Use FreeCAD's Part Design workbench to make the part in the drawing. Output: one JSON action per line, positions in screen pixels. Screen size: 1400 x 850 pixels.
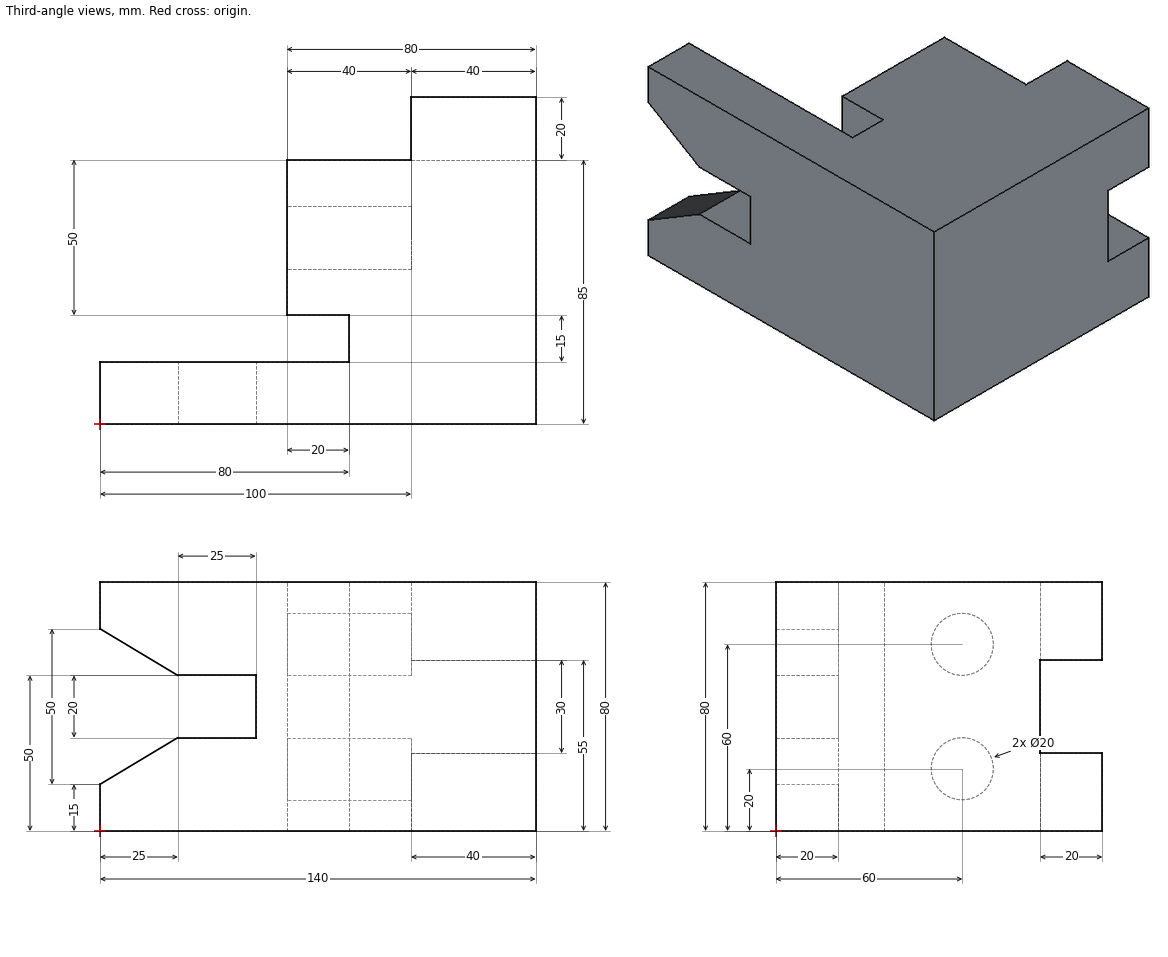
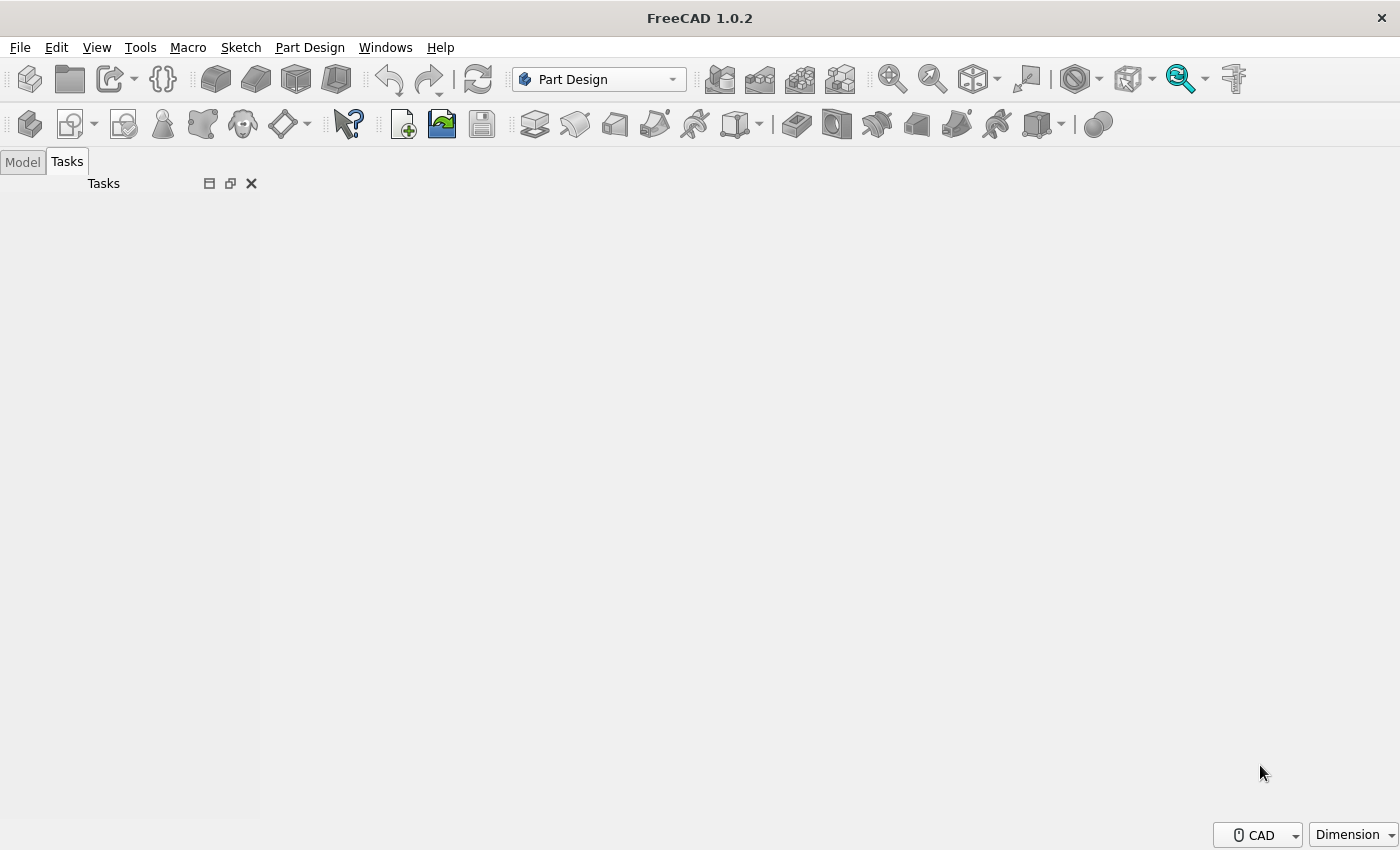
{"action": "key", "text": "ctrl+n"}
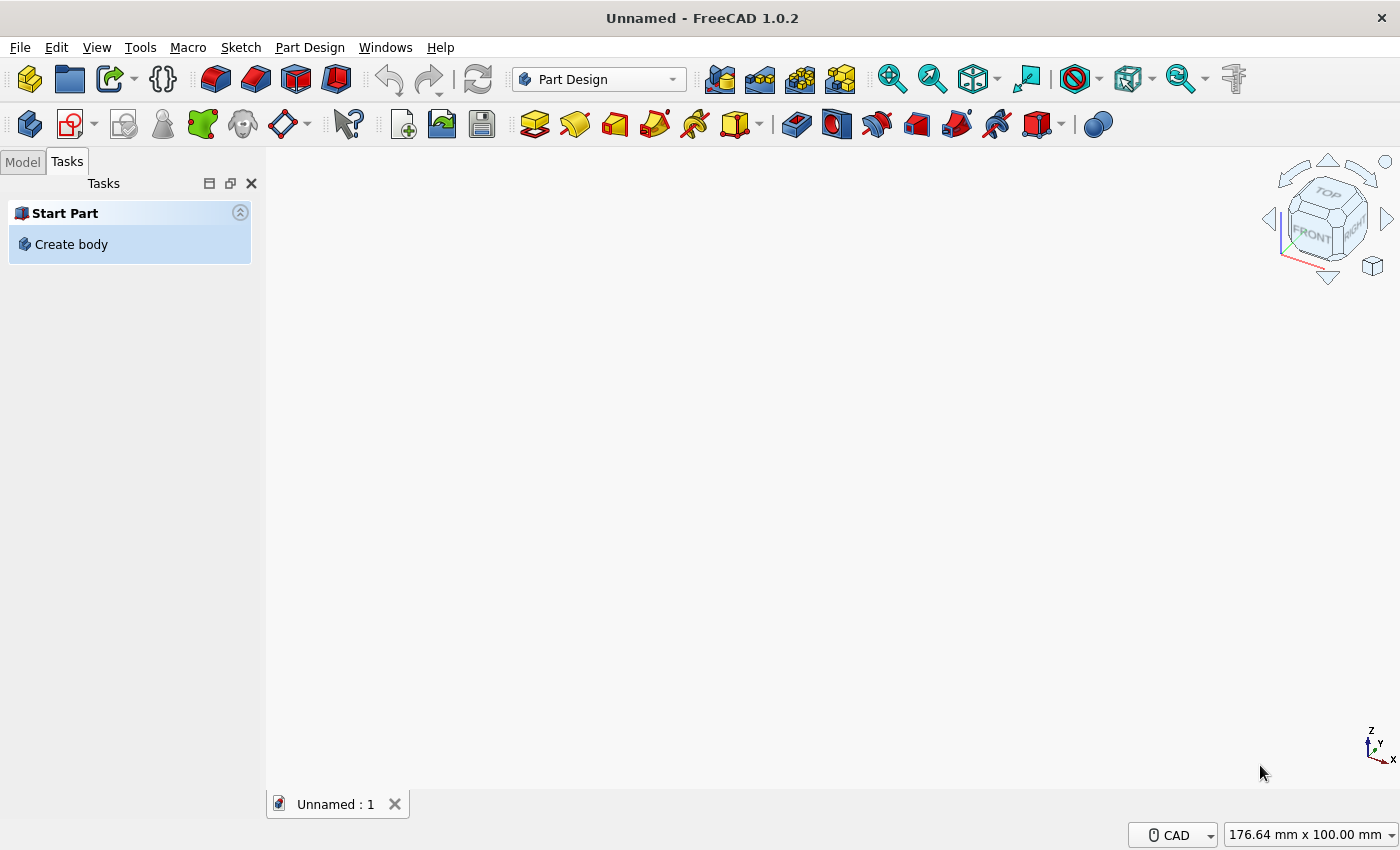
{"action": "left_click", "coordinate": [70, 124]}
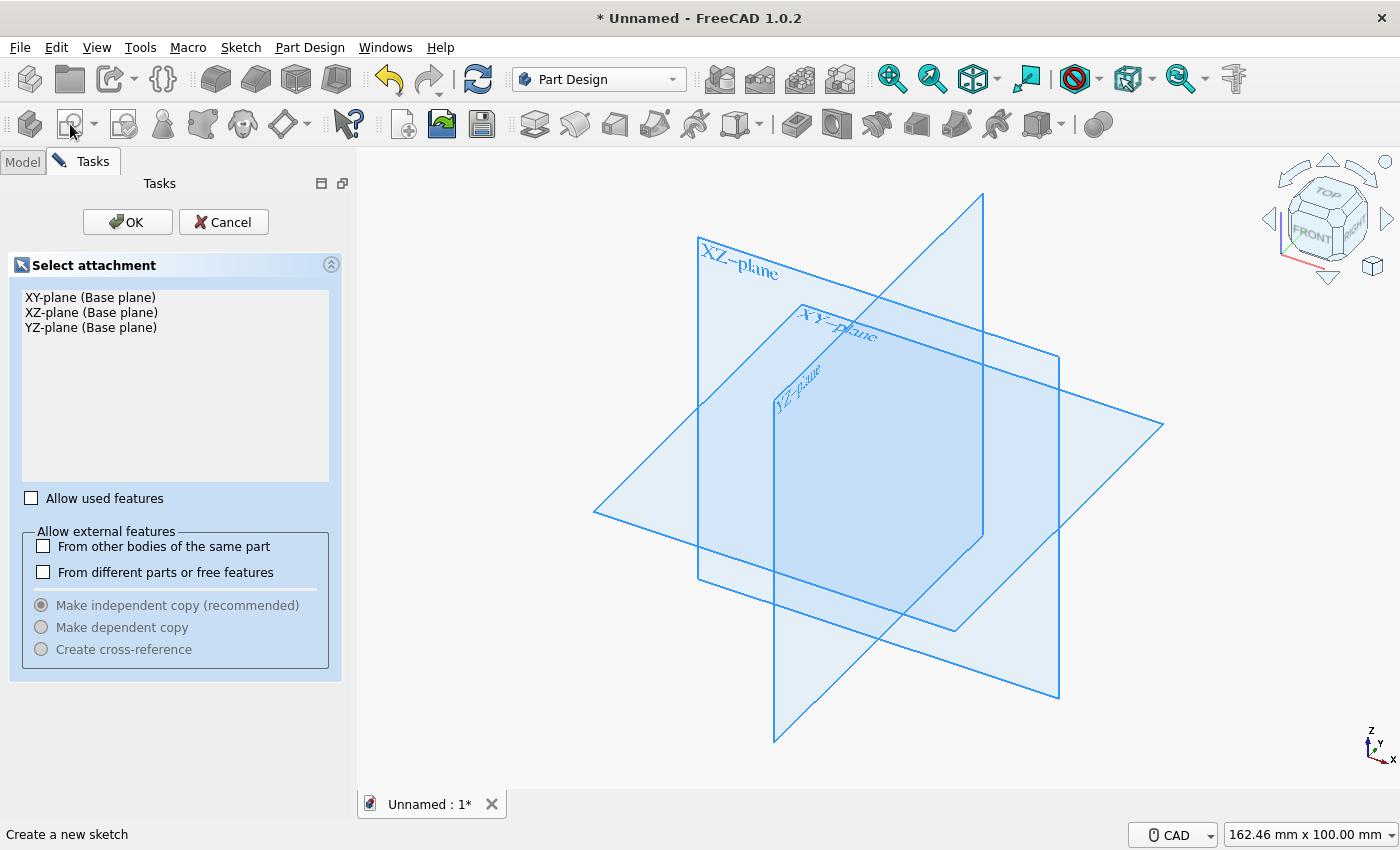
{"action": "left_click", "coordinate": [82, 298]}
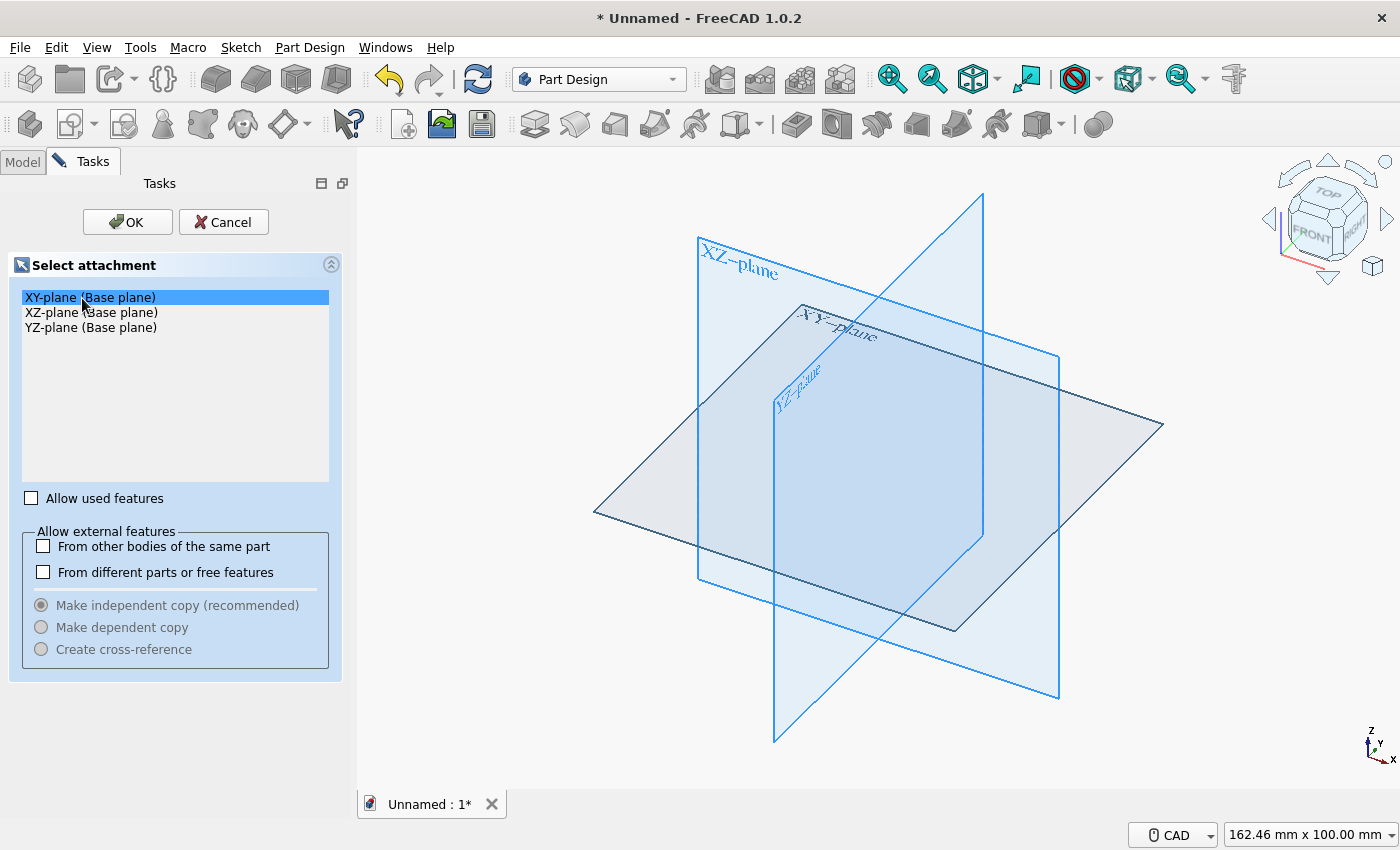
{"action": "left_click", "coordinate": [128, 222]}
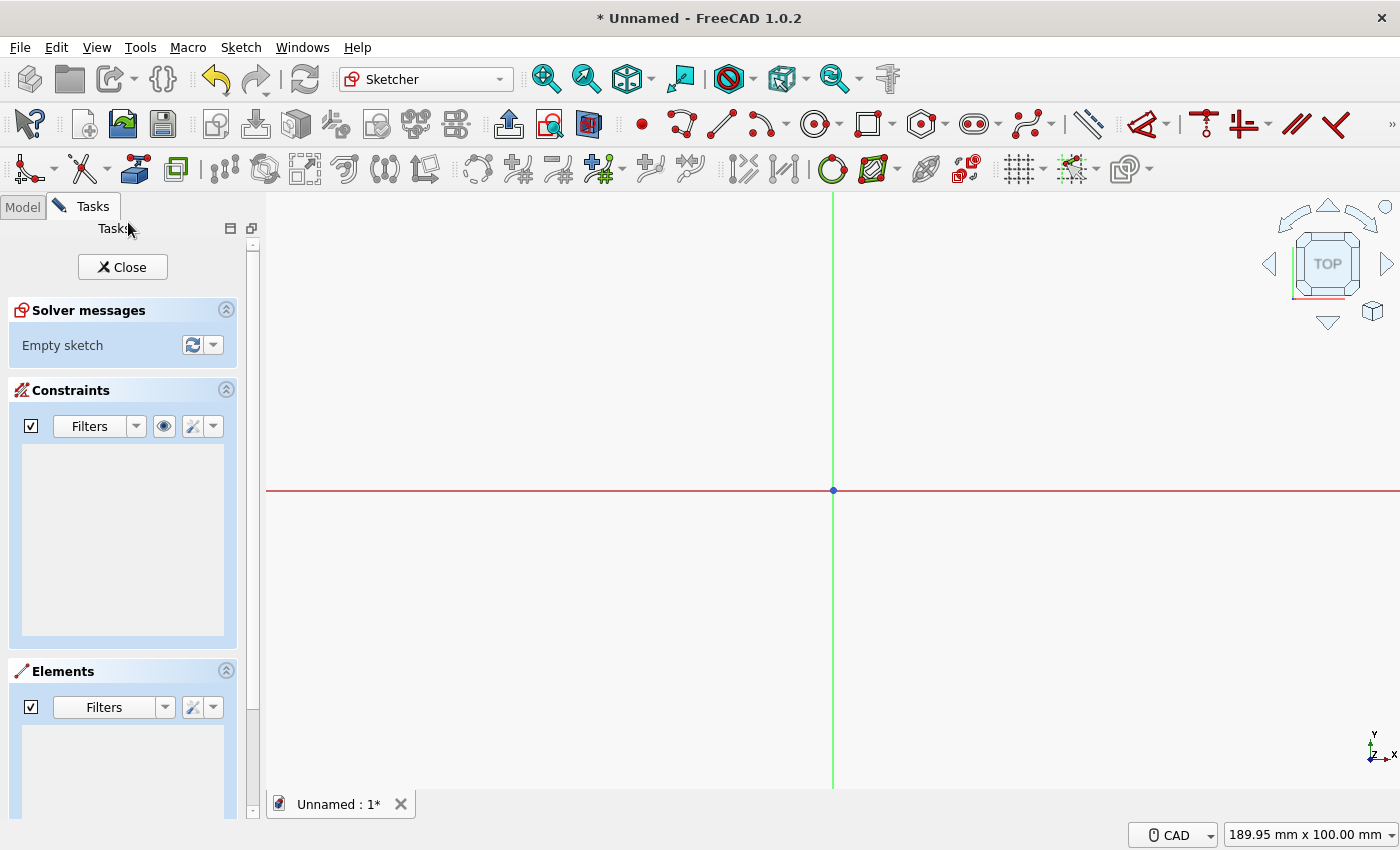
{"action": "scroll", "coordinate": [294, 761], "scroll_direction": "down", "scroll_amount": 3}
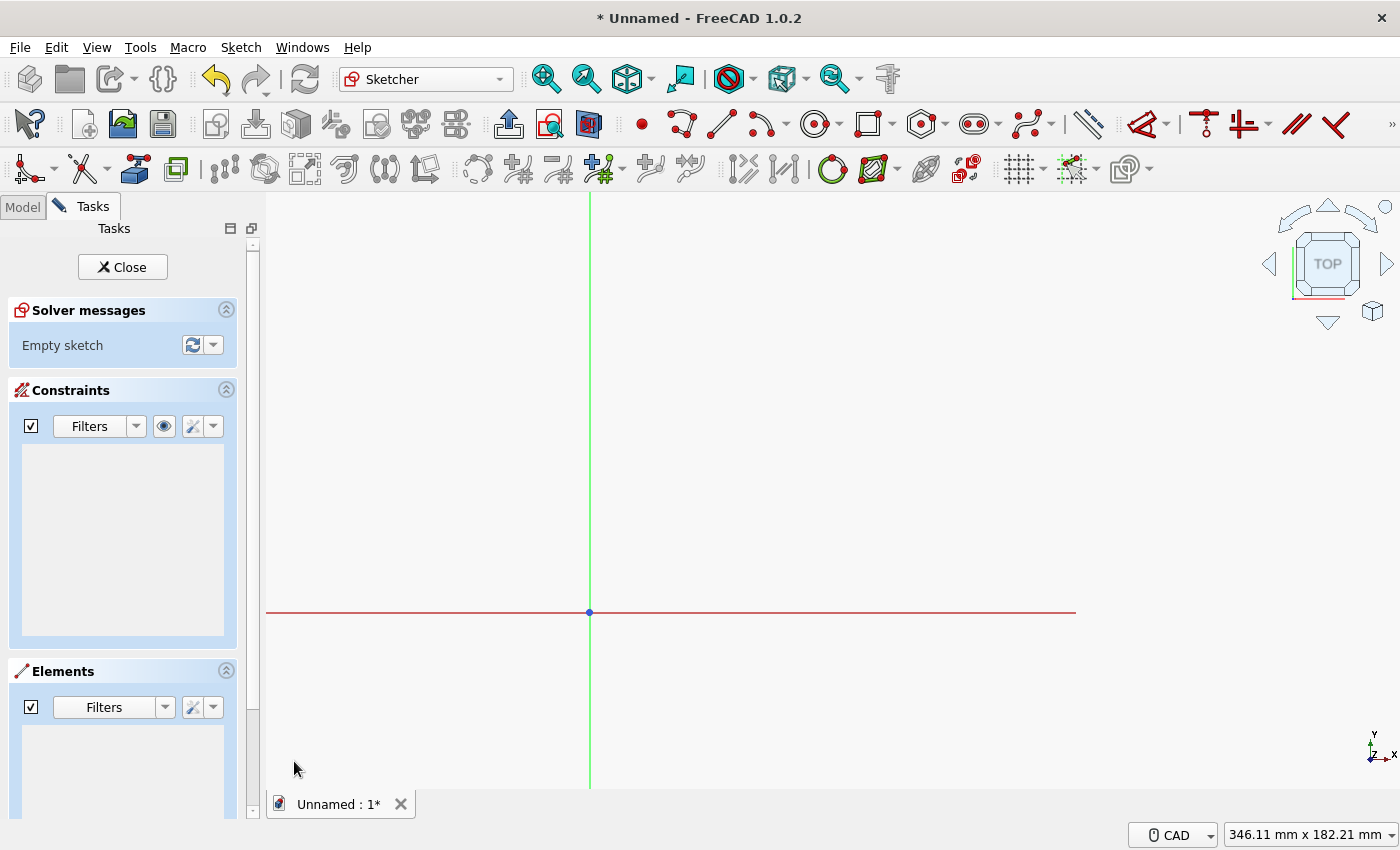
{"action": "scroll", "coordinate": [930, 440], "scroll_direction": "up", "scroll_amount": 2}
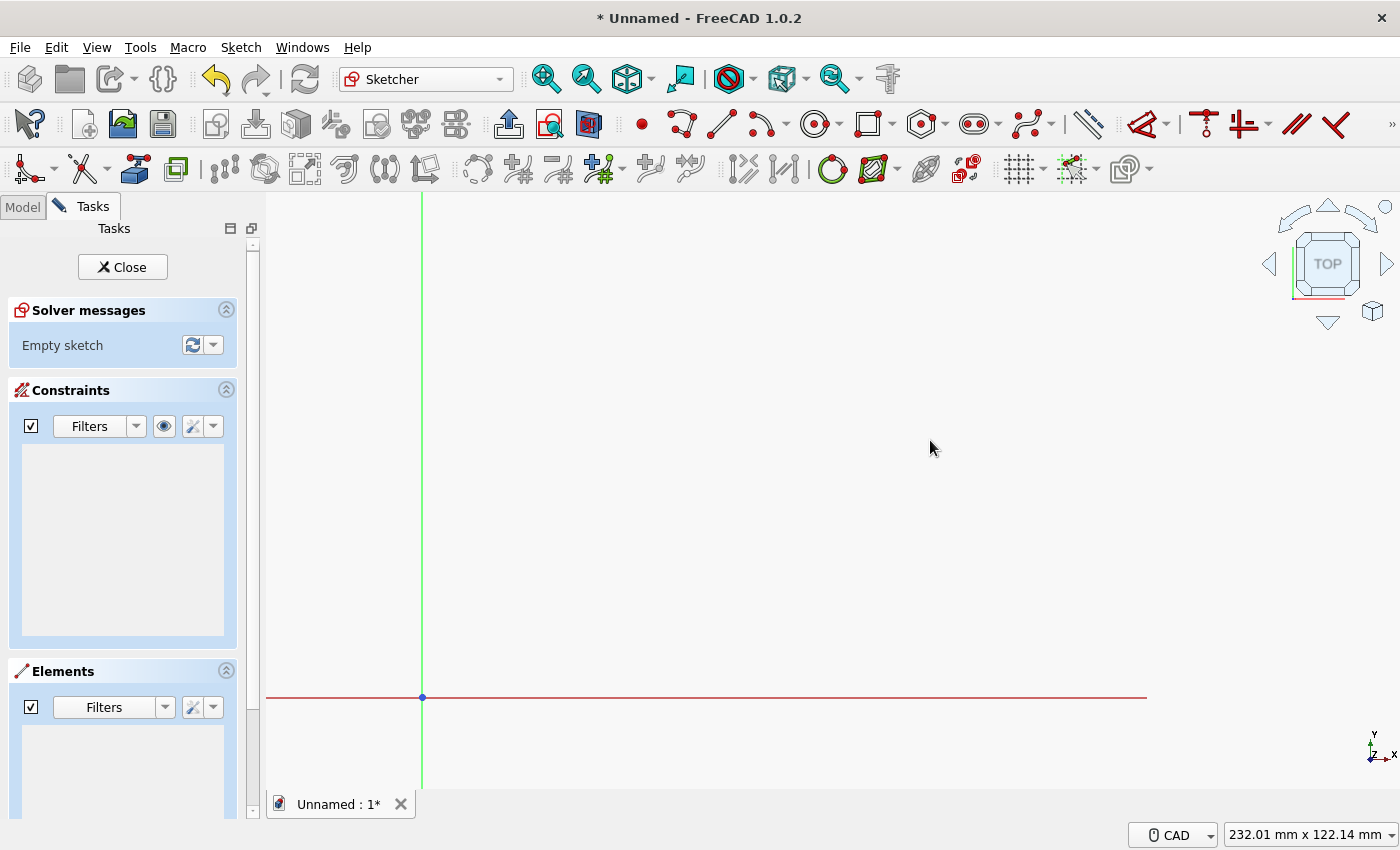
{"action": "left_click", "coordinate": [682, 124]}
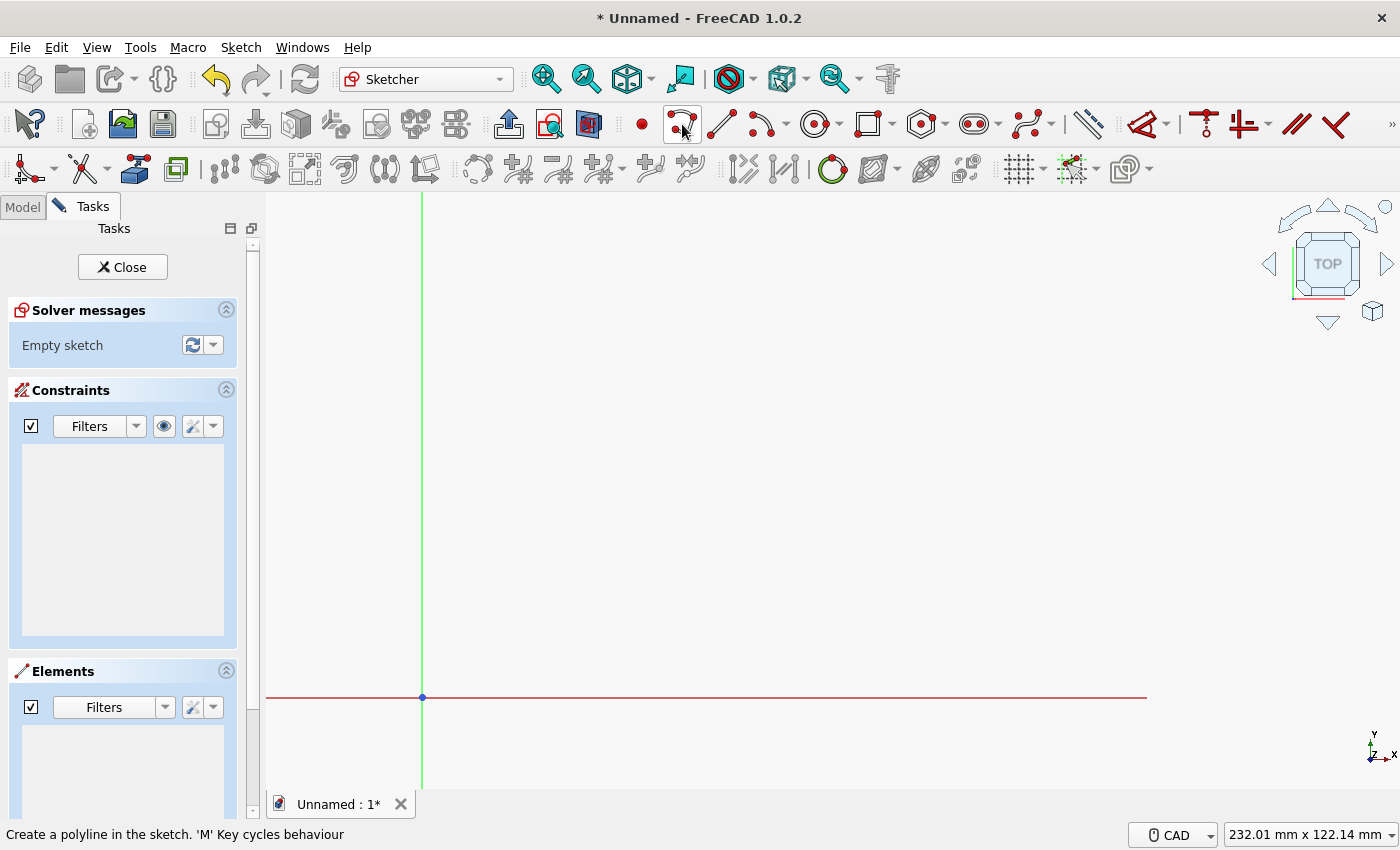
{"action": "left_click", "coordinate": [422, 698]}
{"action": "left_click", "coordinate": [1107, 689]}
{"action": "left_click", "coordinate": [1107, 282]}
{"action": "left_click", "coordinate": [715, 282]}
{"action": "left_click", "coordinate": [715, 527]}
{"action": "left_click", "coordinate": [813, 527]}
{"action": "left_click", "coordinate": [813, 600]}
{"action": "left_click", "coordinate": [431, 600]}
{"action": "left_click", "coordinate": [422, 698]}
{"action": "key", "text": "Escape"}
{"action": "key", "text": "Escape"}